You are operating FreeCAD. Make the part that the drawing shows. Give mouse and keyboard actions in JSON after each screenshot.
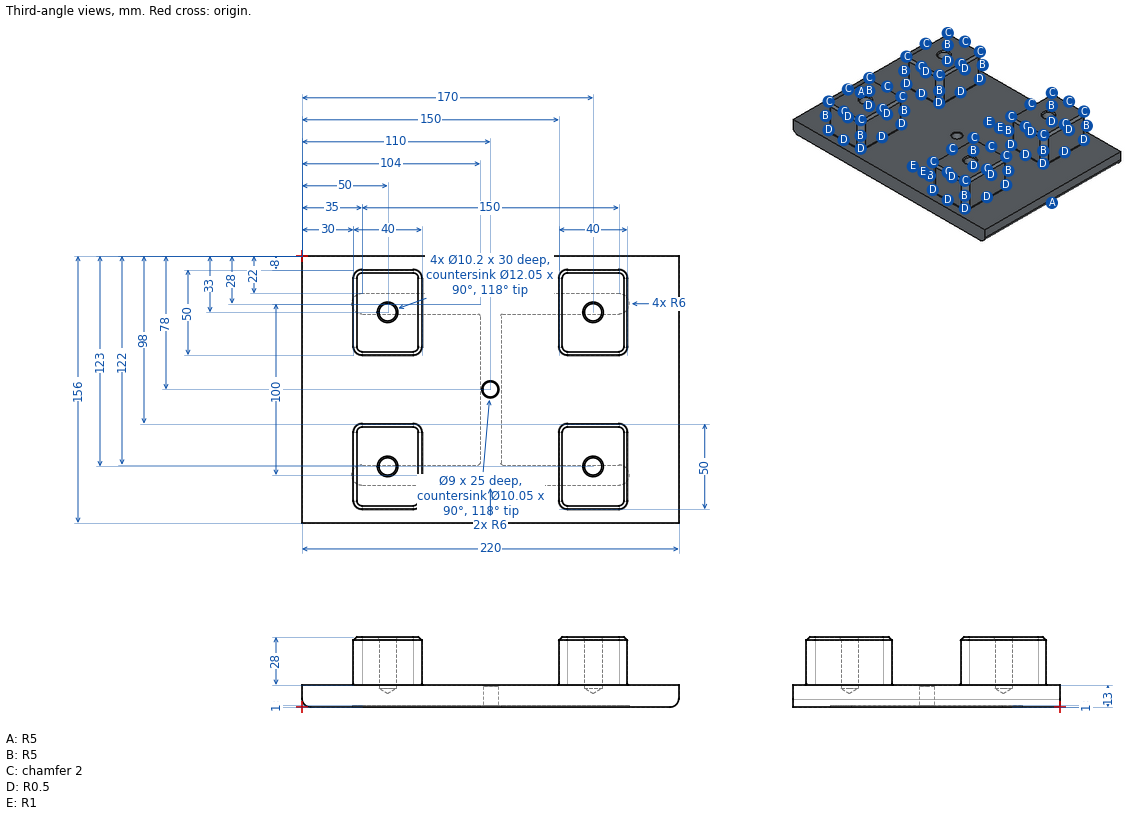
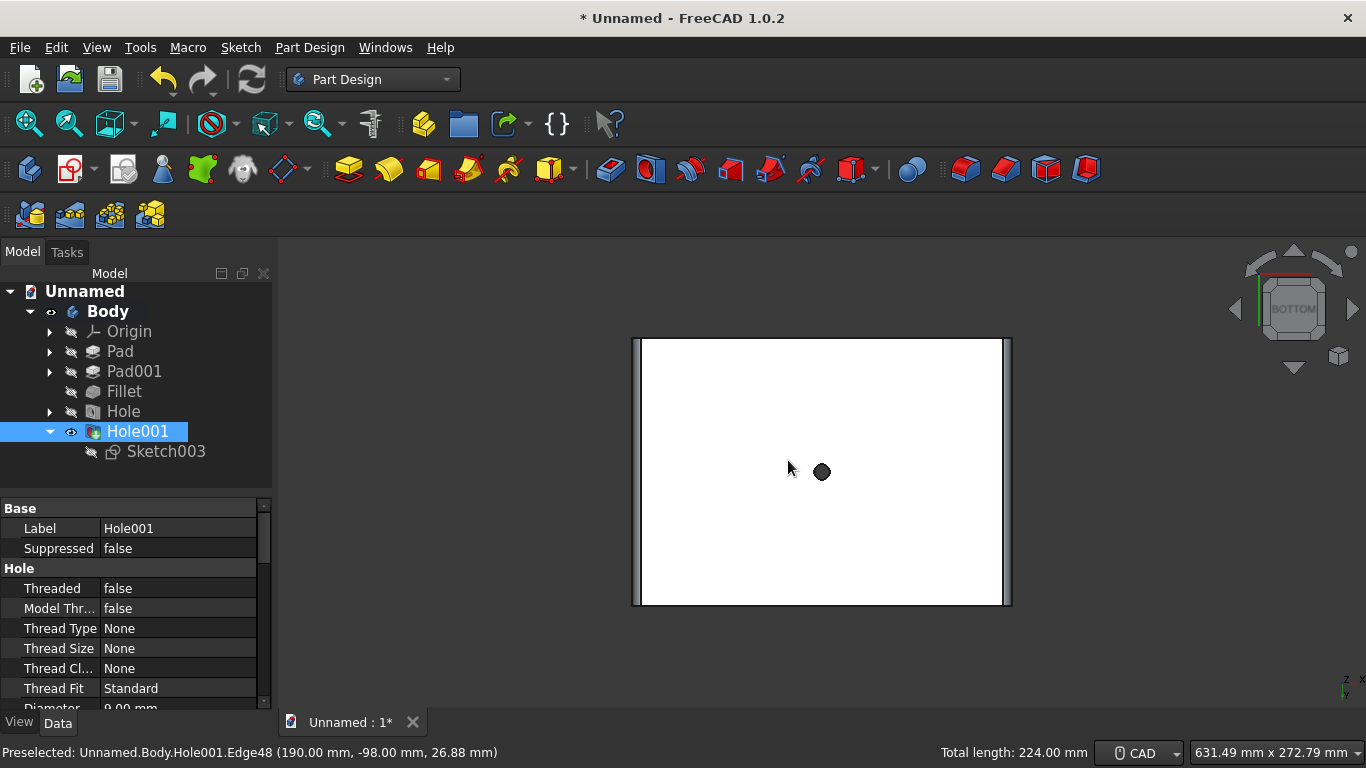
{"action": "key", "text": "4"}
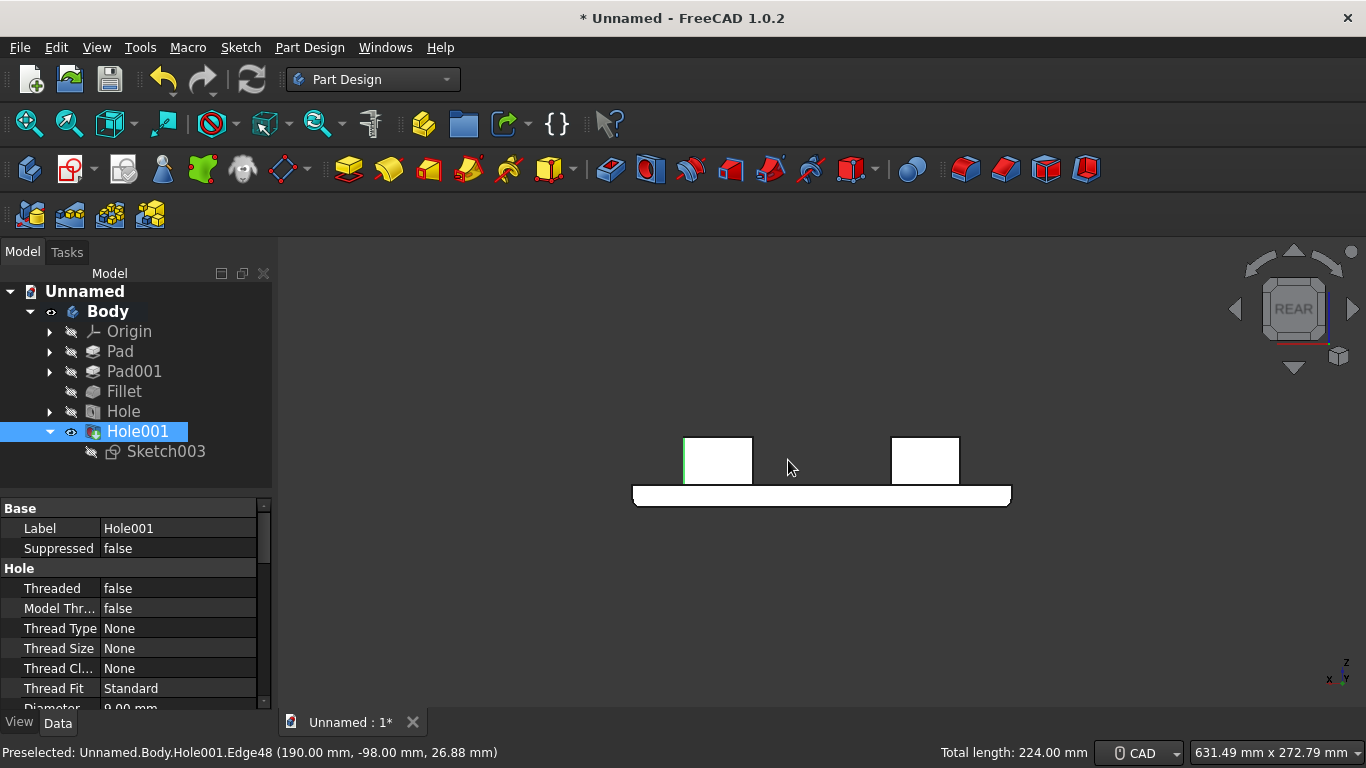
{"action": "key", "text": "v f"}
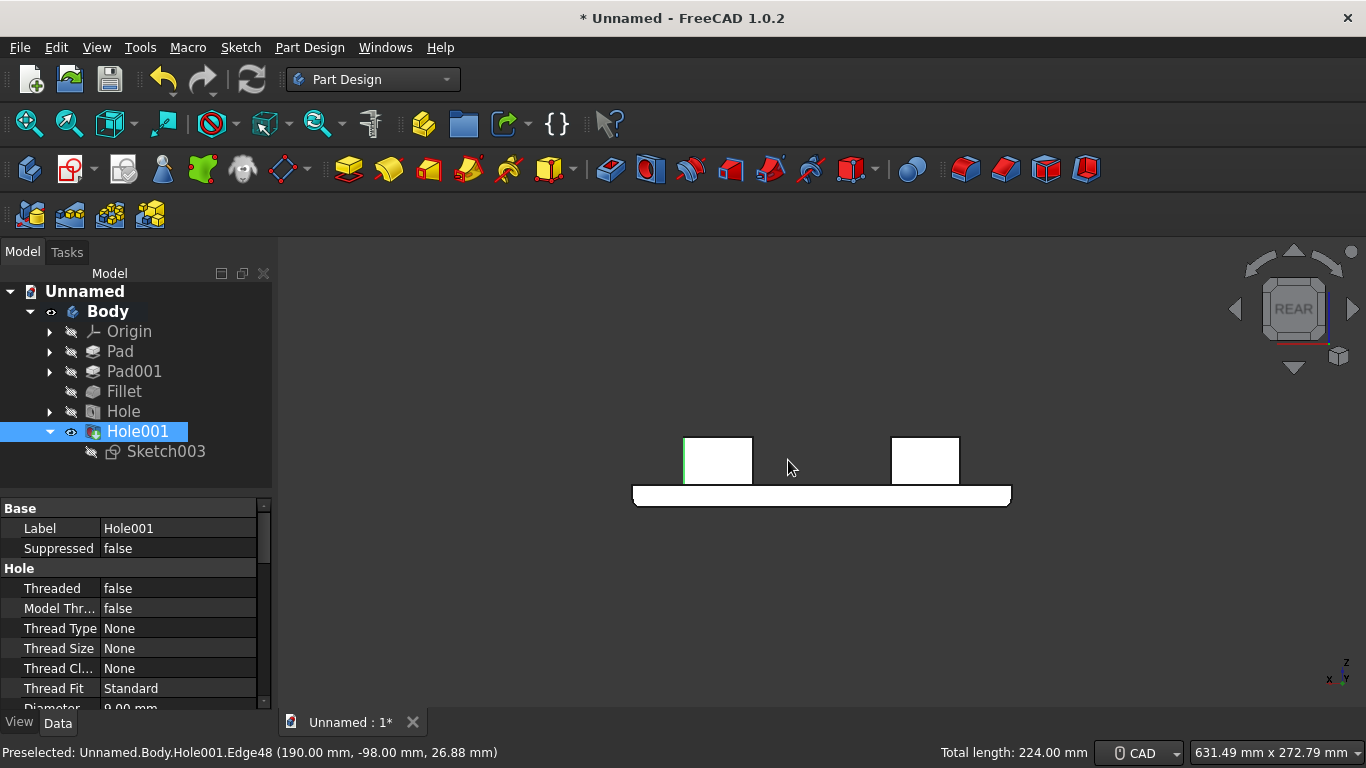
{"action": "left_click", "coordinate": [891, 460], "text": "ctrl"}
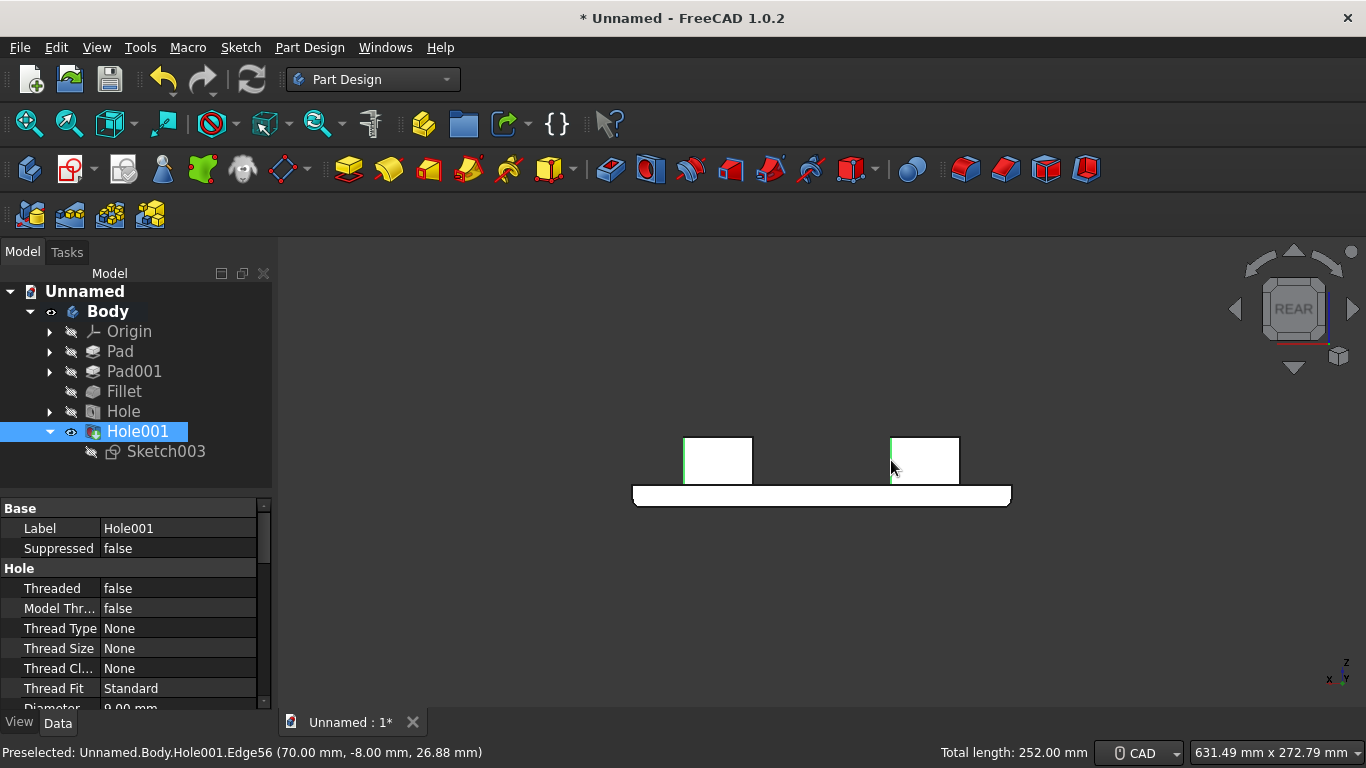
{"action": "left_click", "coordinate": [960, 460], "text": "ctrl"}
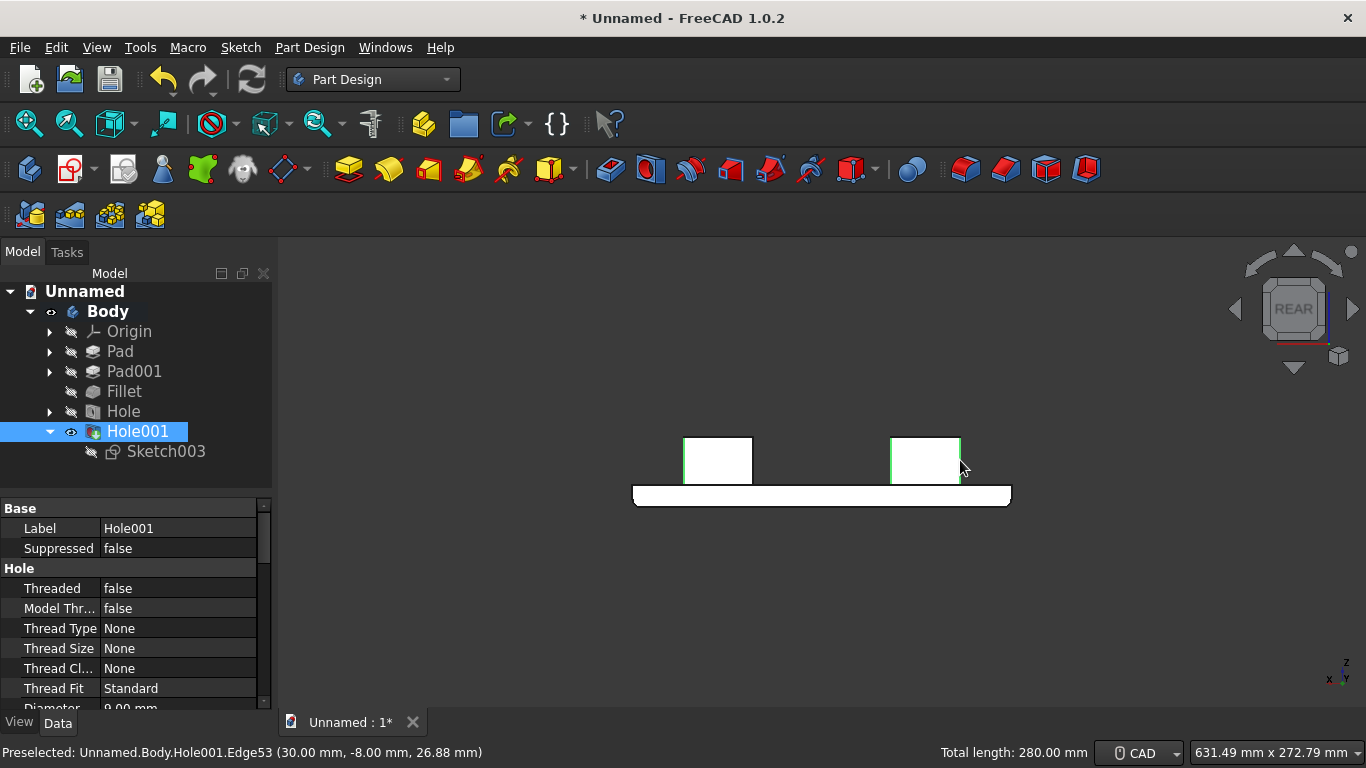
{"action": "left_click", "coordinate": [753, 460], "text": "ctrl"}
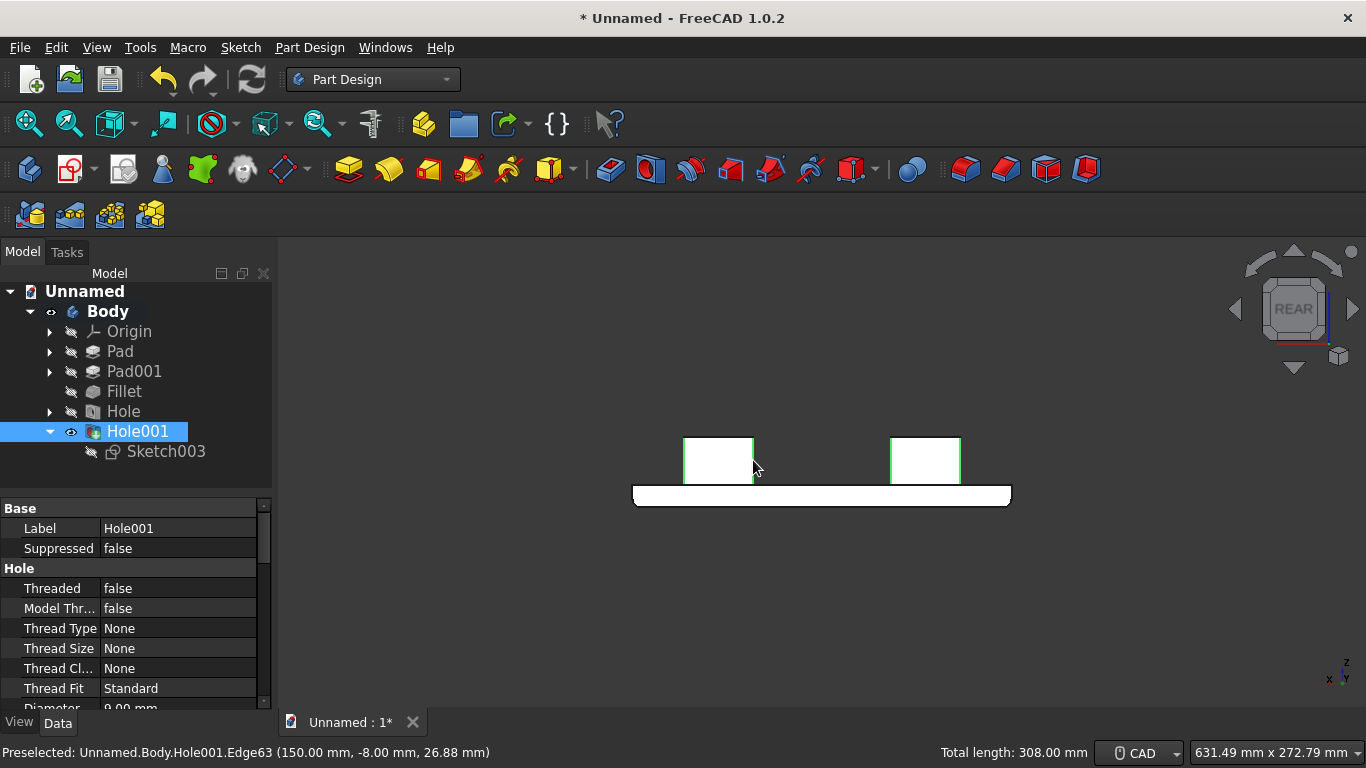
{"action": "key", "text": "6"}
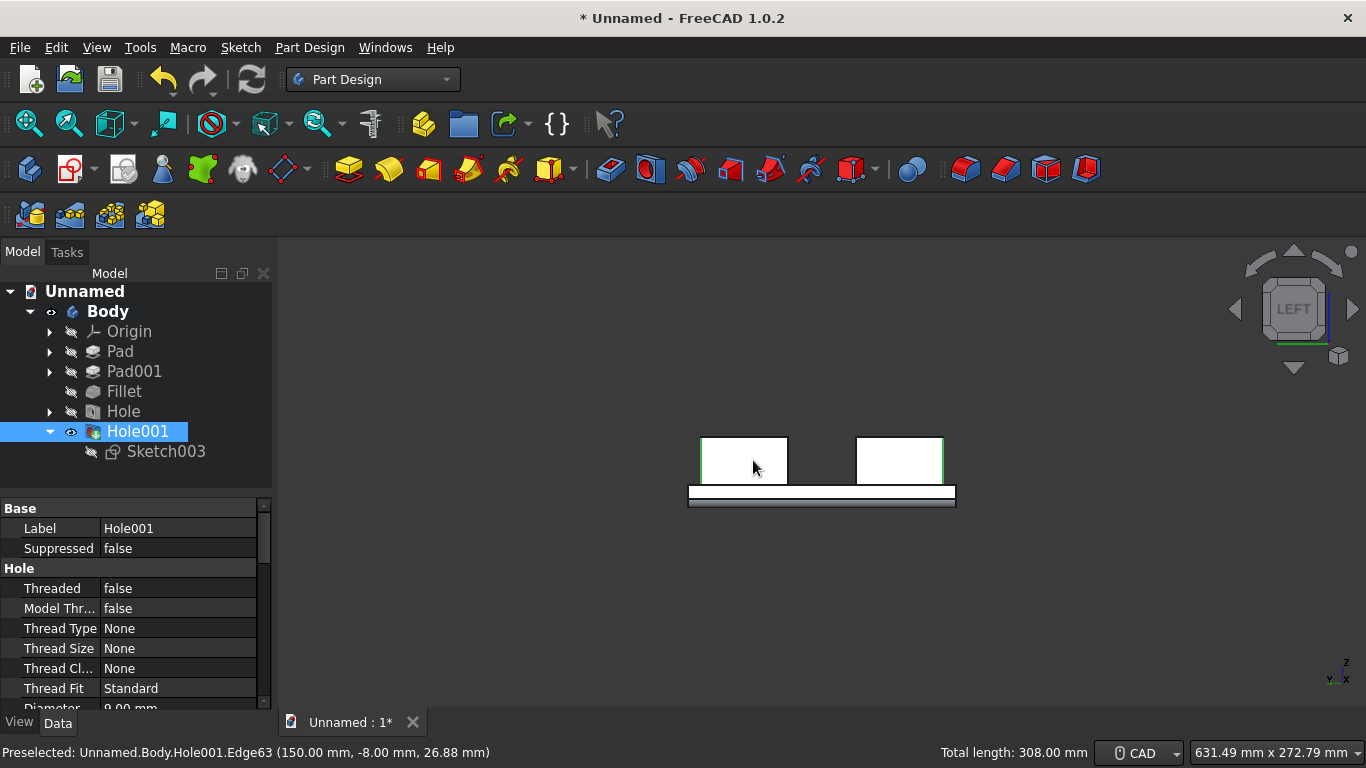
{"action": "left_click", "coordinate": [30, 124]}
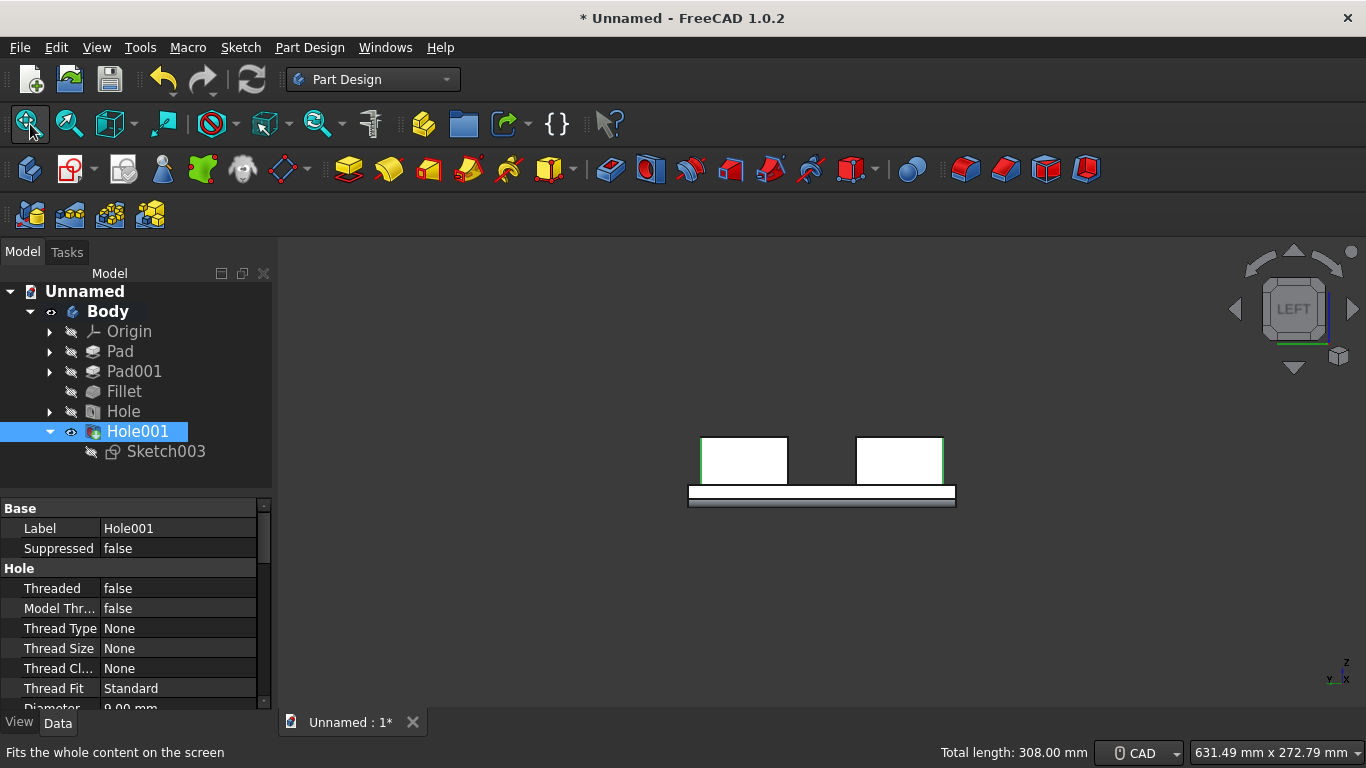
{"action": "left_click", "coordinate": [788, 460], "text": "ctrl"}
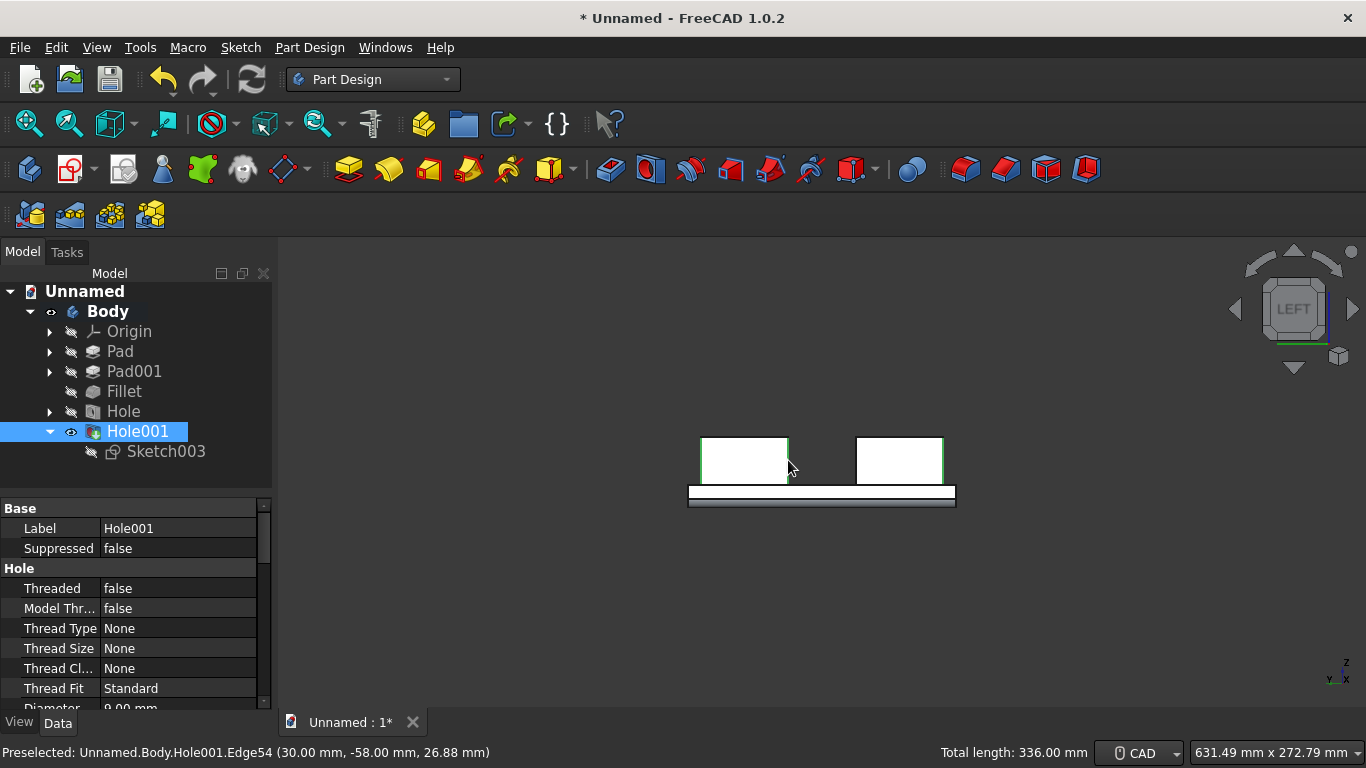
{"action": "left_click", "coordinate": [856, 460], "text": "ctrl"}